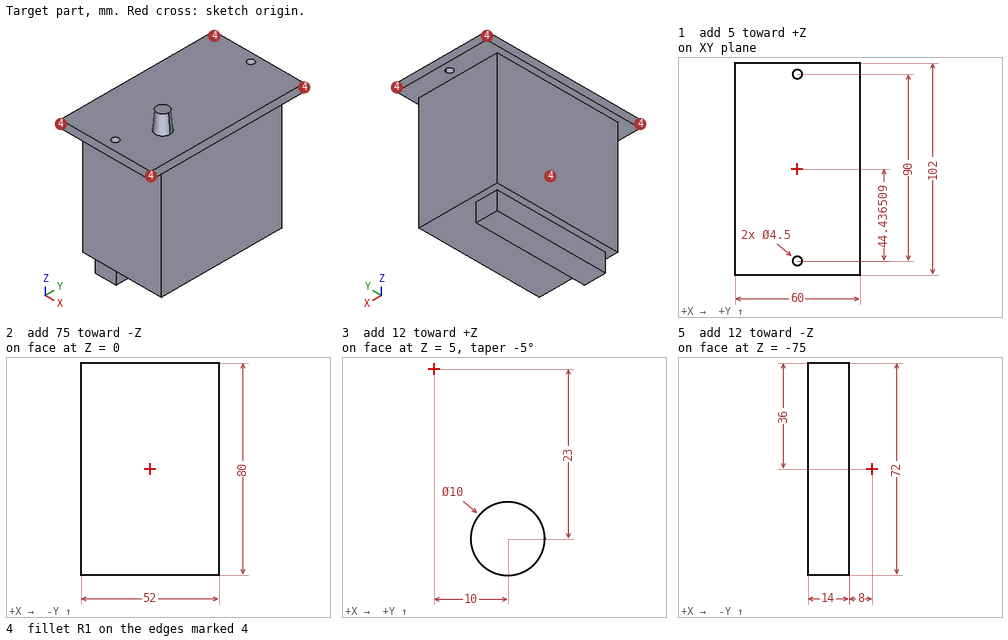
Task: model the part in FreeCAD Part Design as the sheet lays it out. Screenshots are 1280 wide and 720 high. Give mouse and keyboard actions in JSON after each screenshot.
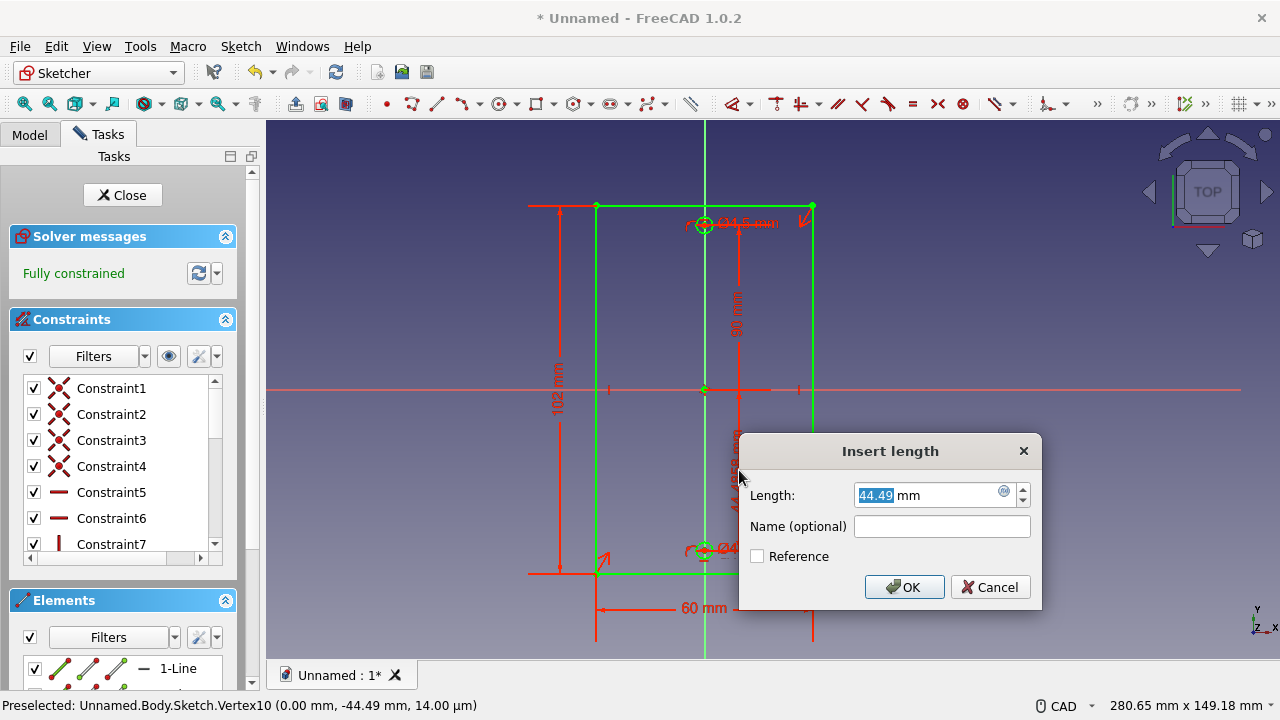
{"action": "type", "text": "44.436509"}
{"action": "key", "text": "Return"}
{"action": "key", "text": "Escape"}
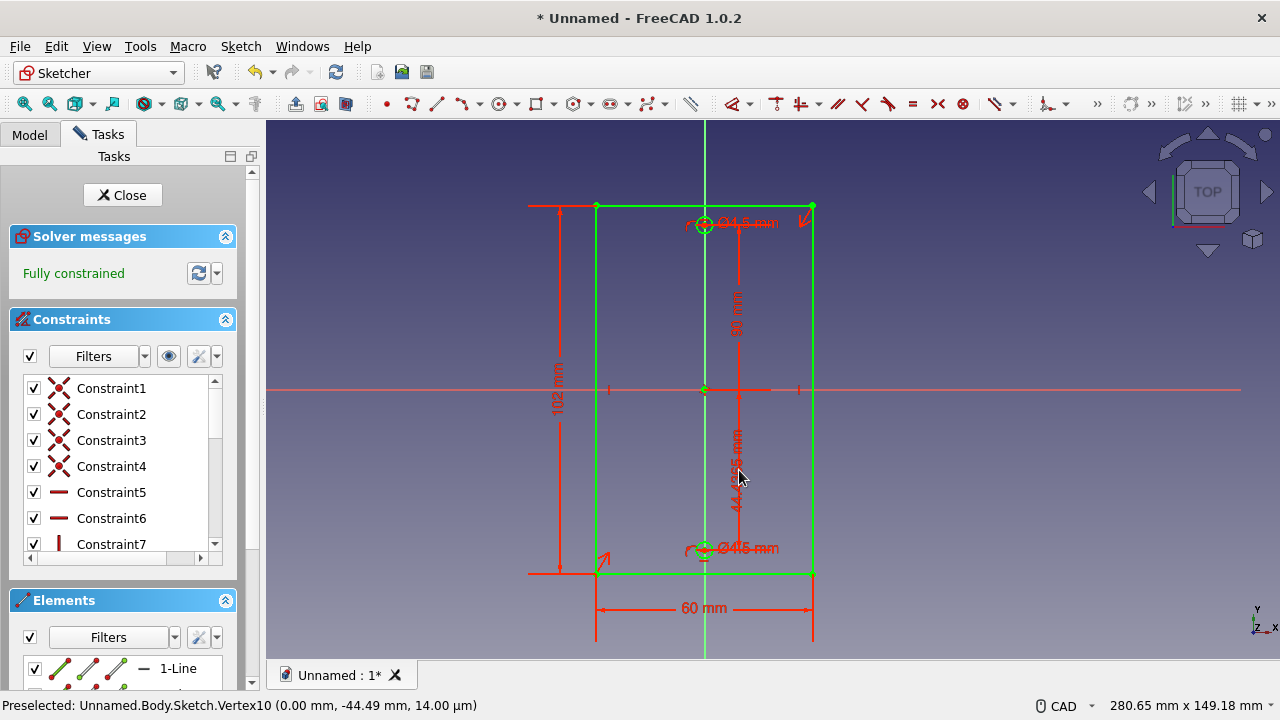
{"action": "left_click", "coordinate": [123, 195]}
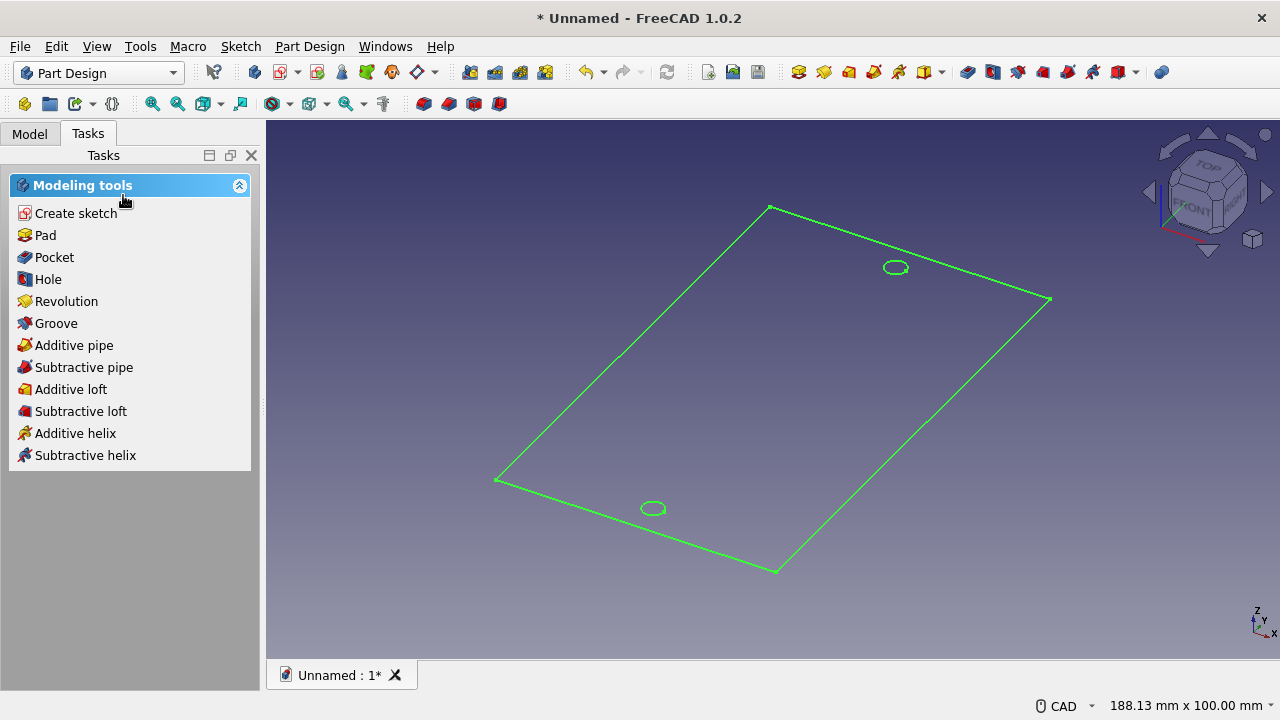
{"action": "left_click", "coordinate": [799, 72]}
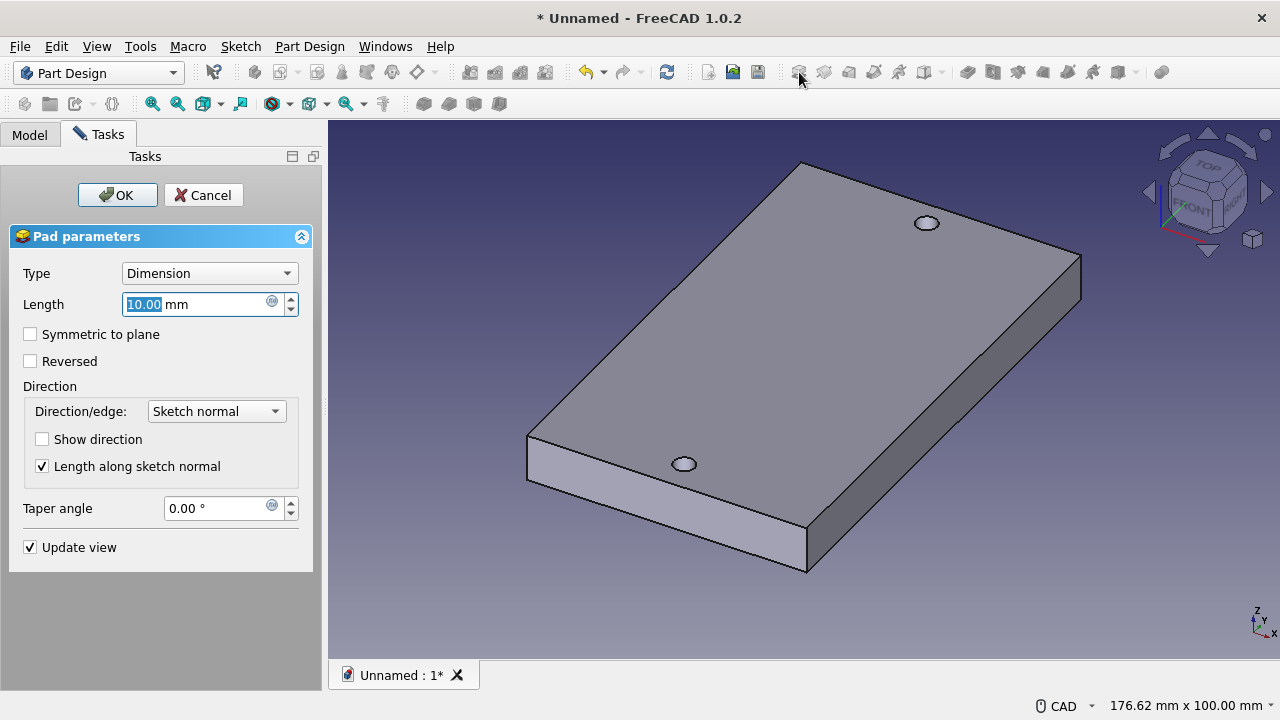
{"action": "type", "text": "5"}
{"action": "key", "text": "Tab"}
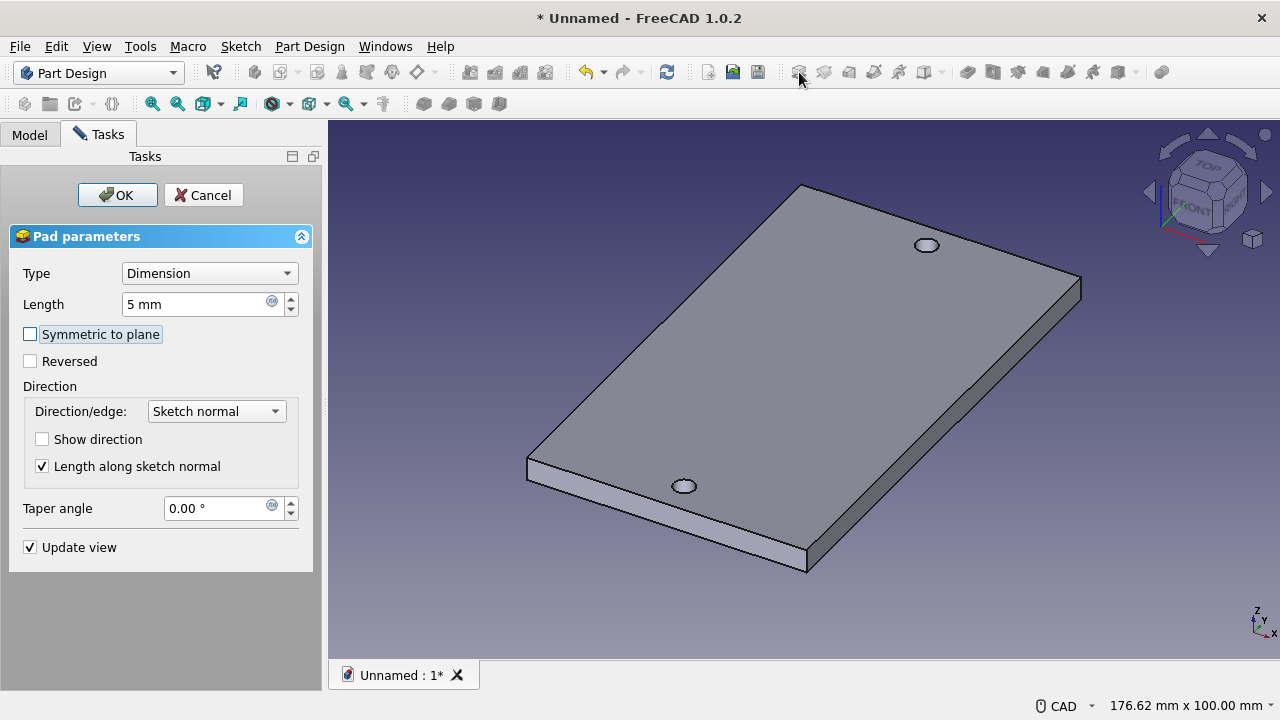
{"action": "left_click", "coordinate": [118, 195]}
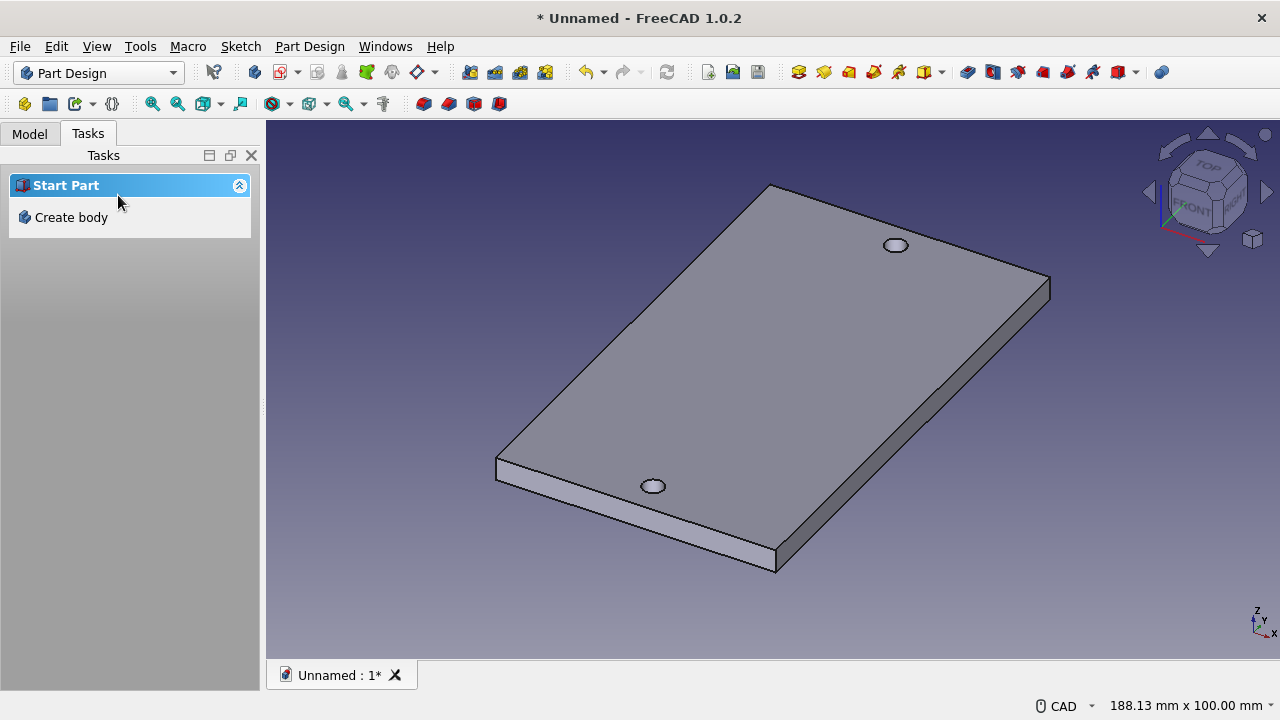
{"action": "key", "text": "5"}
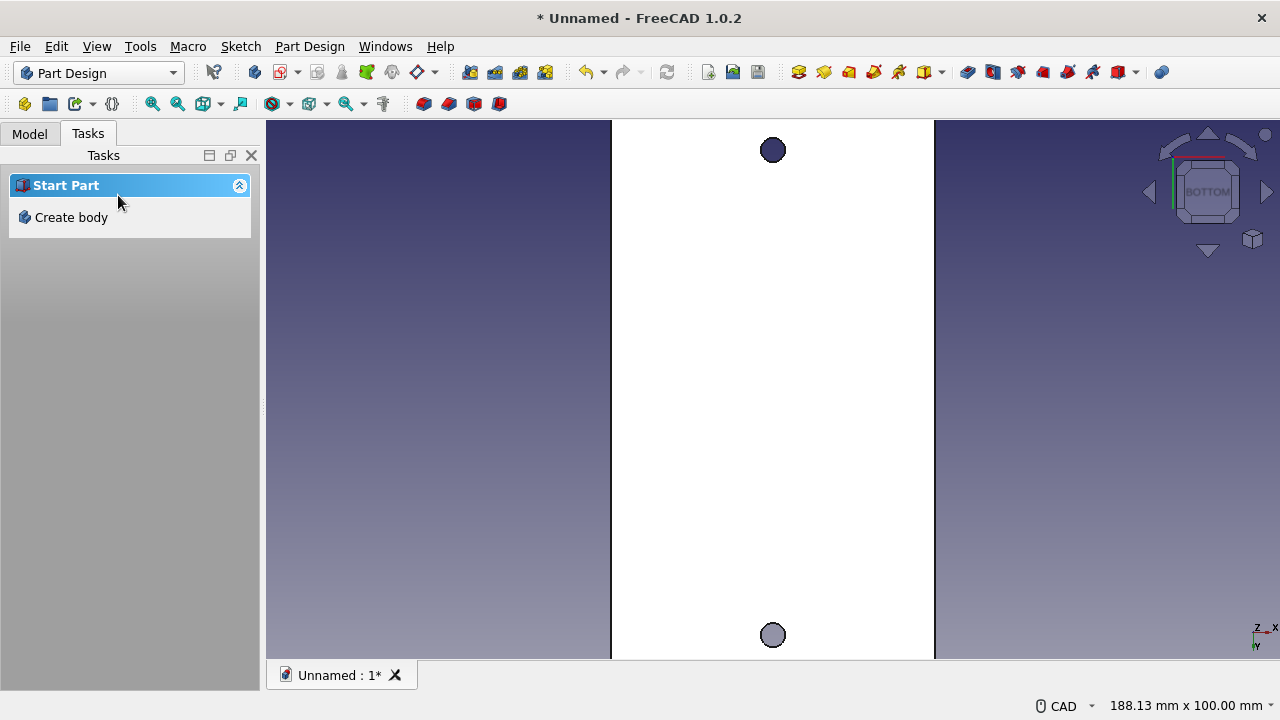
{"action": "key", "text": "v f"}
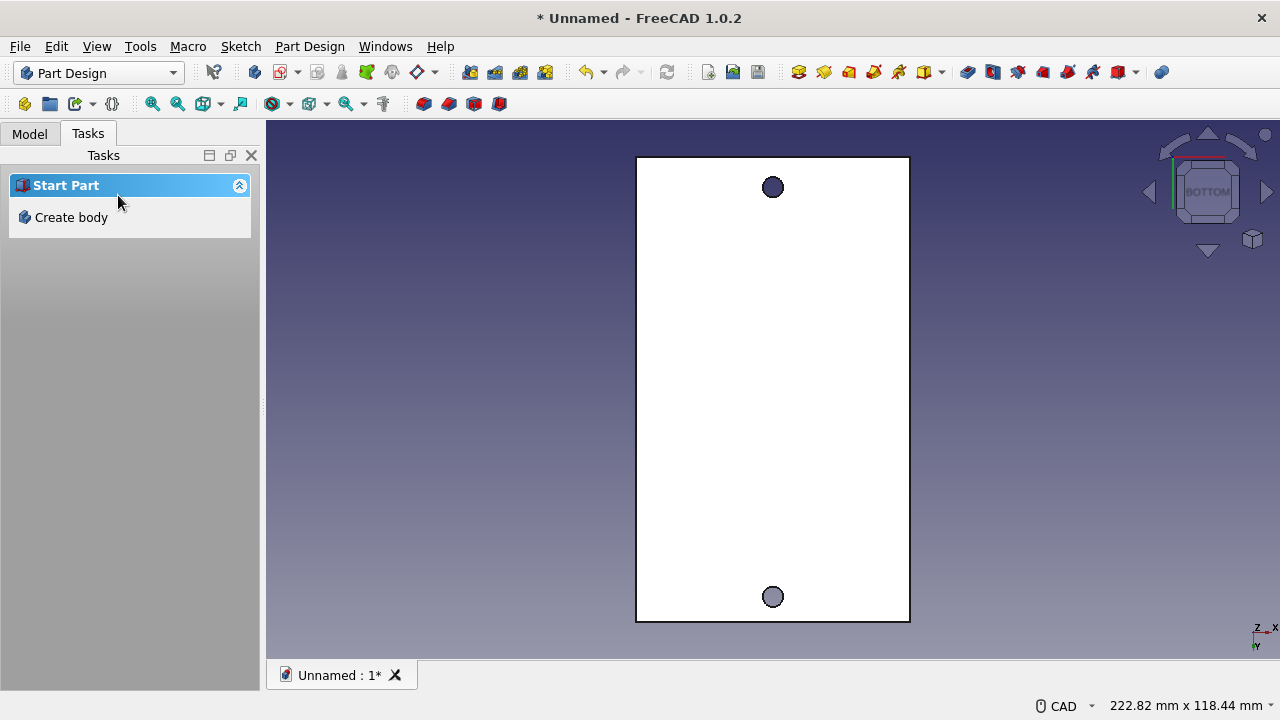
{"action": "left_click", "coordinate": [773, 388]}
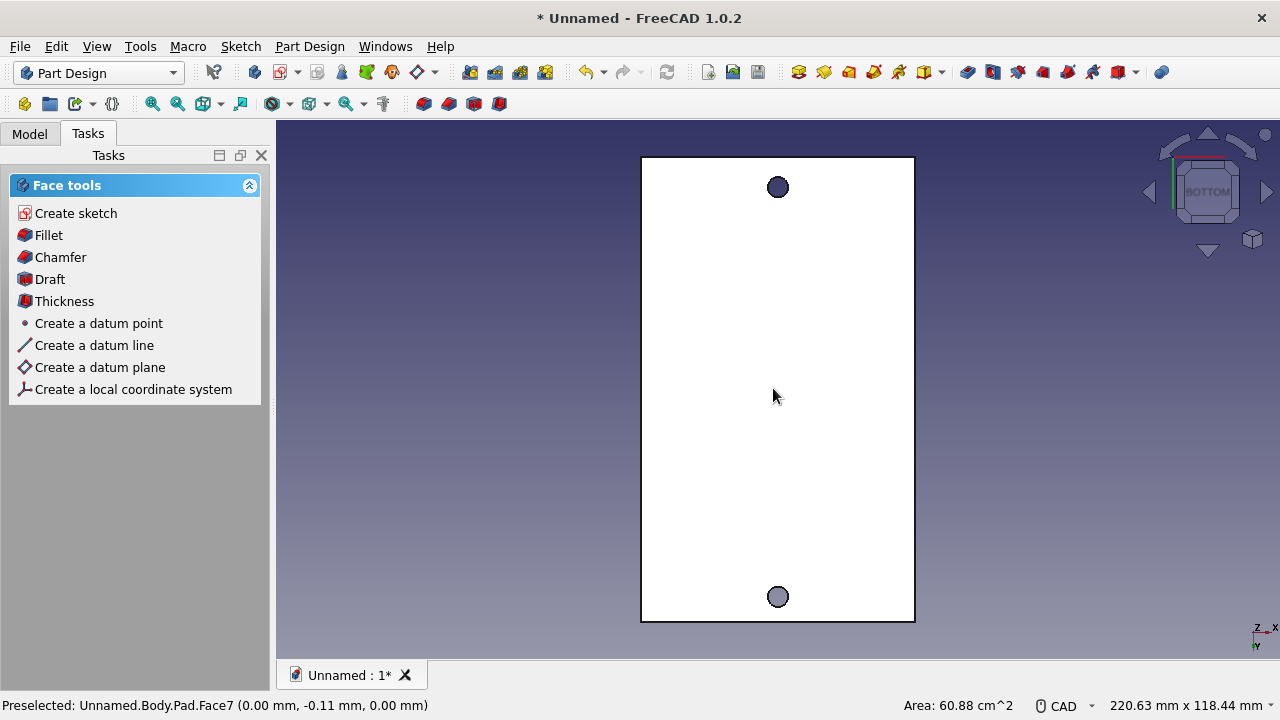
{"action": "left_click", "coordinate": [280, 72]}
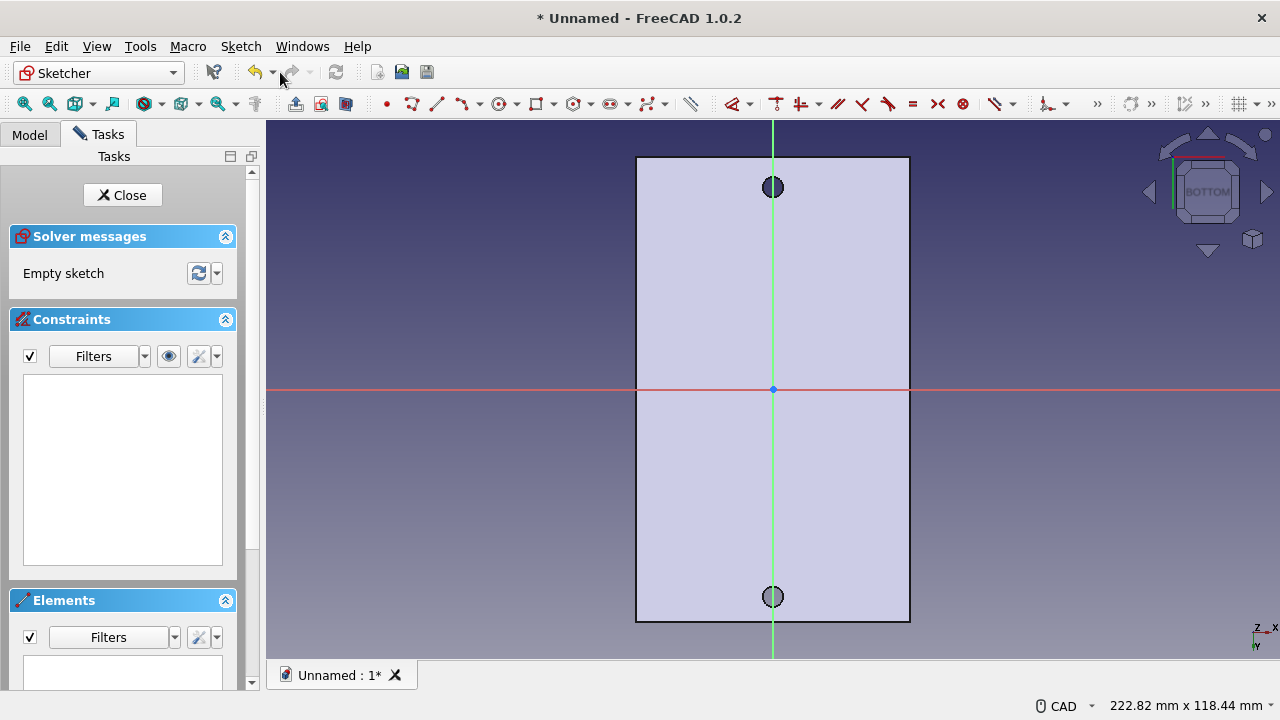
{"action": "key", "text": "g v"}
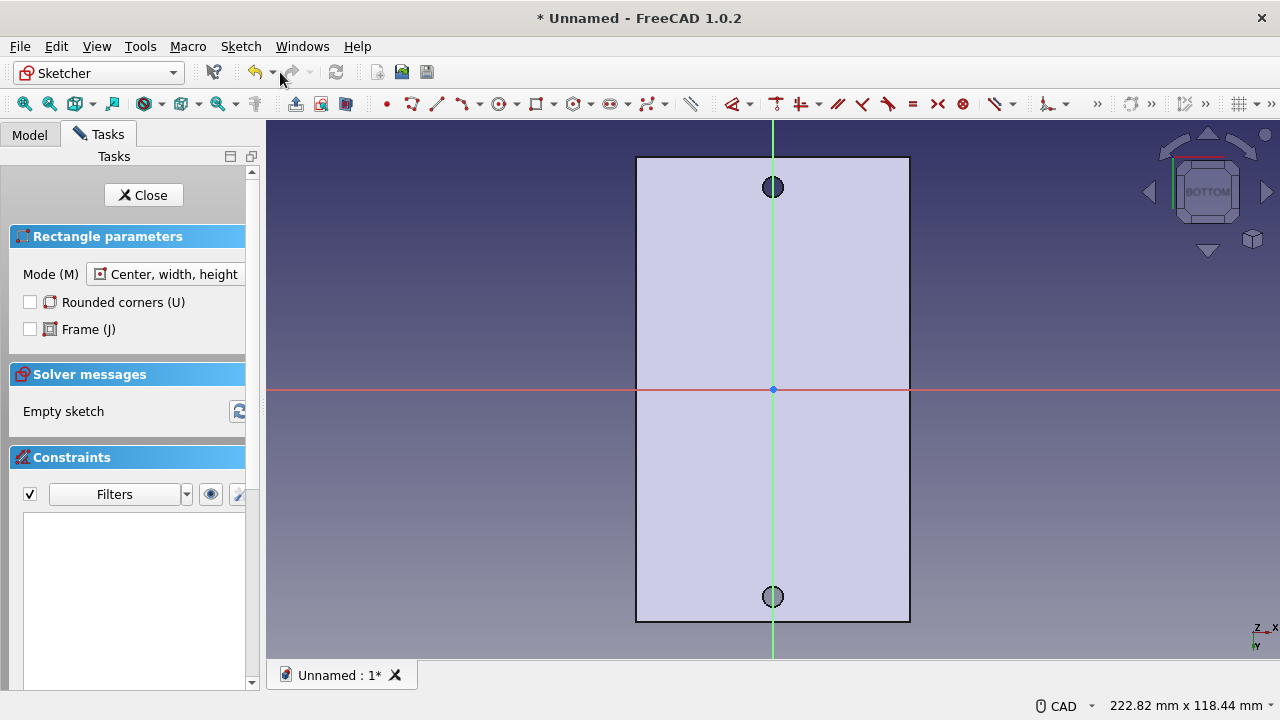
{"action": "left_click", "coordinate": [773, 390]}
{"action": "mouse_move", "coordinate": [891, 207]}